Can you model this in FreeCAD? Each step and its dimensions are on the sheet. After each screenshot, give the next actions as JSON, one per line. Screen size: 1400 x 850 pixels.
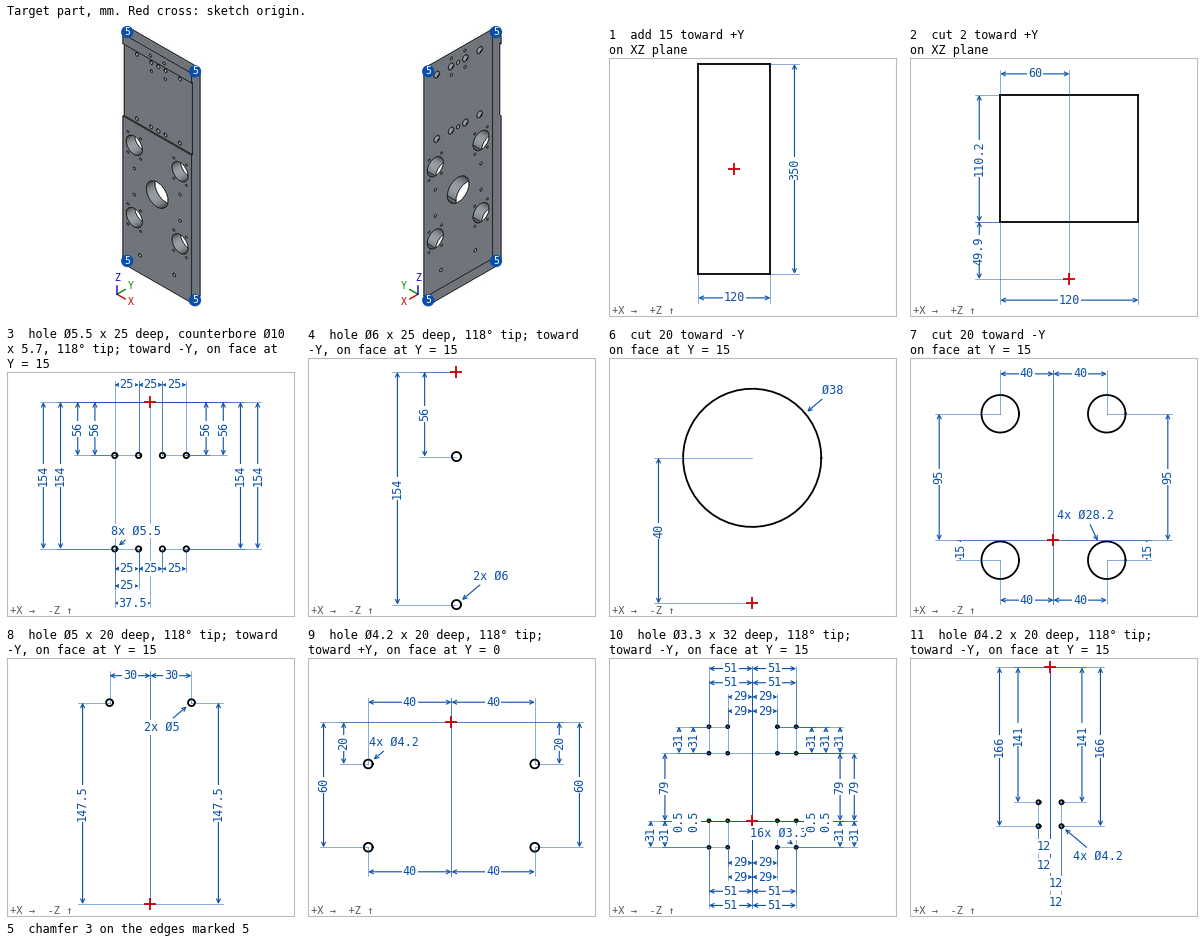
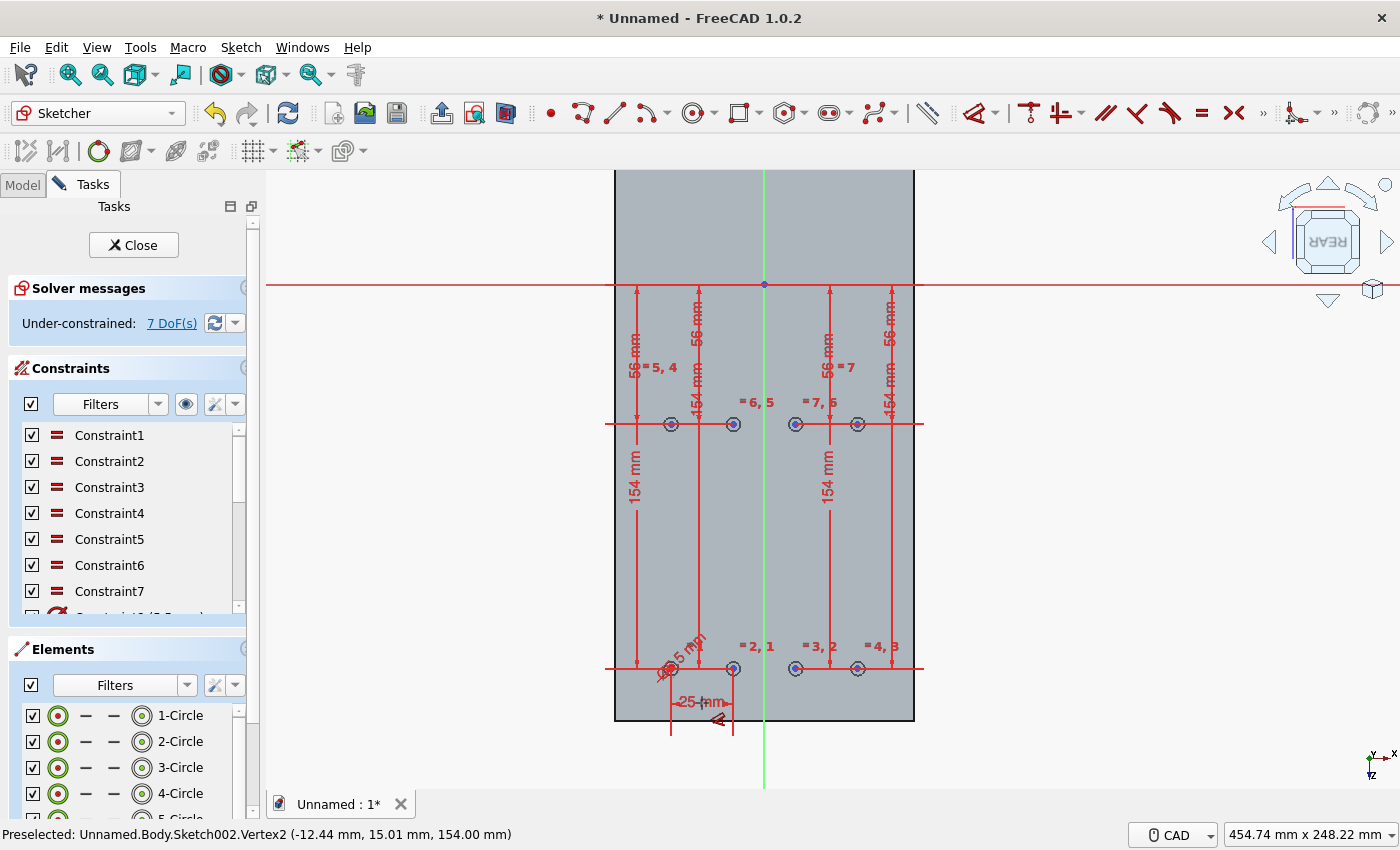
{"action": "left_click", "coordinate": [733, 669]}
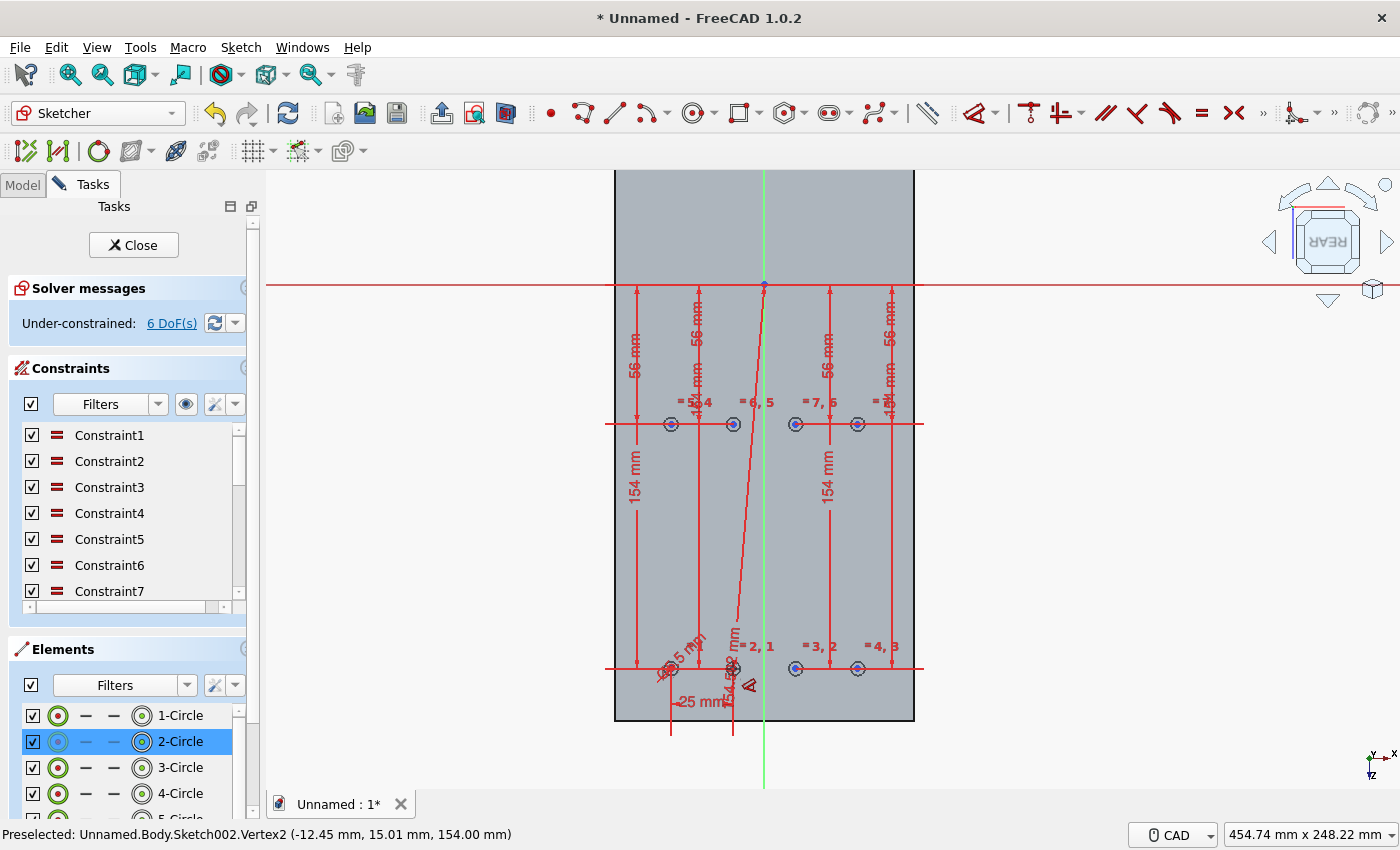
{"action": "left_click", "coordinate": [796, 669]}
{"action": "left_click", "coordinate": [779, 703]}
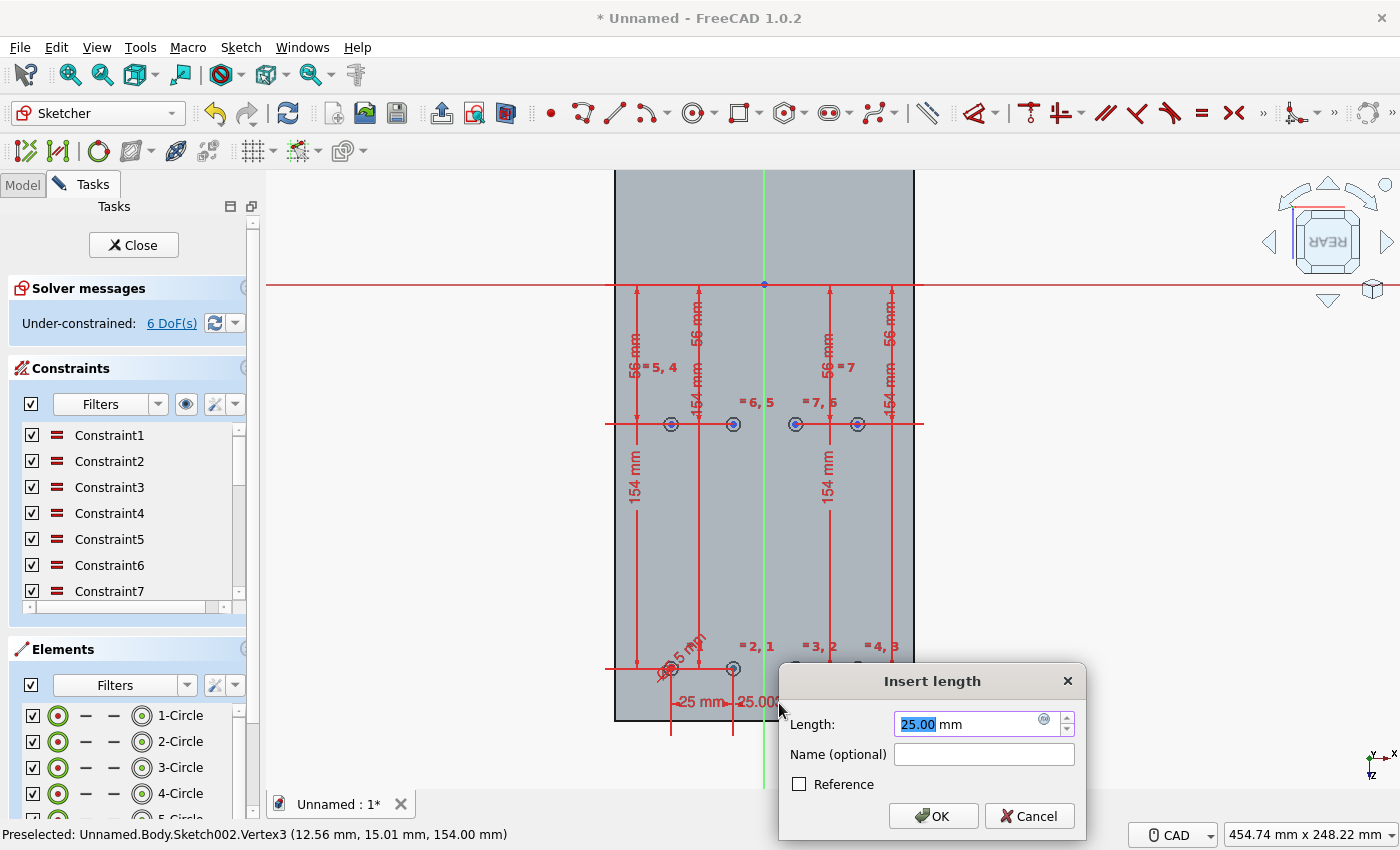
{"action": "type", "text": "25"}
{"action": "key", "text": "Return"}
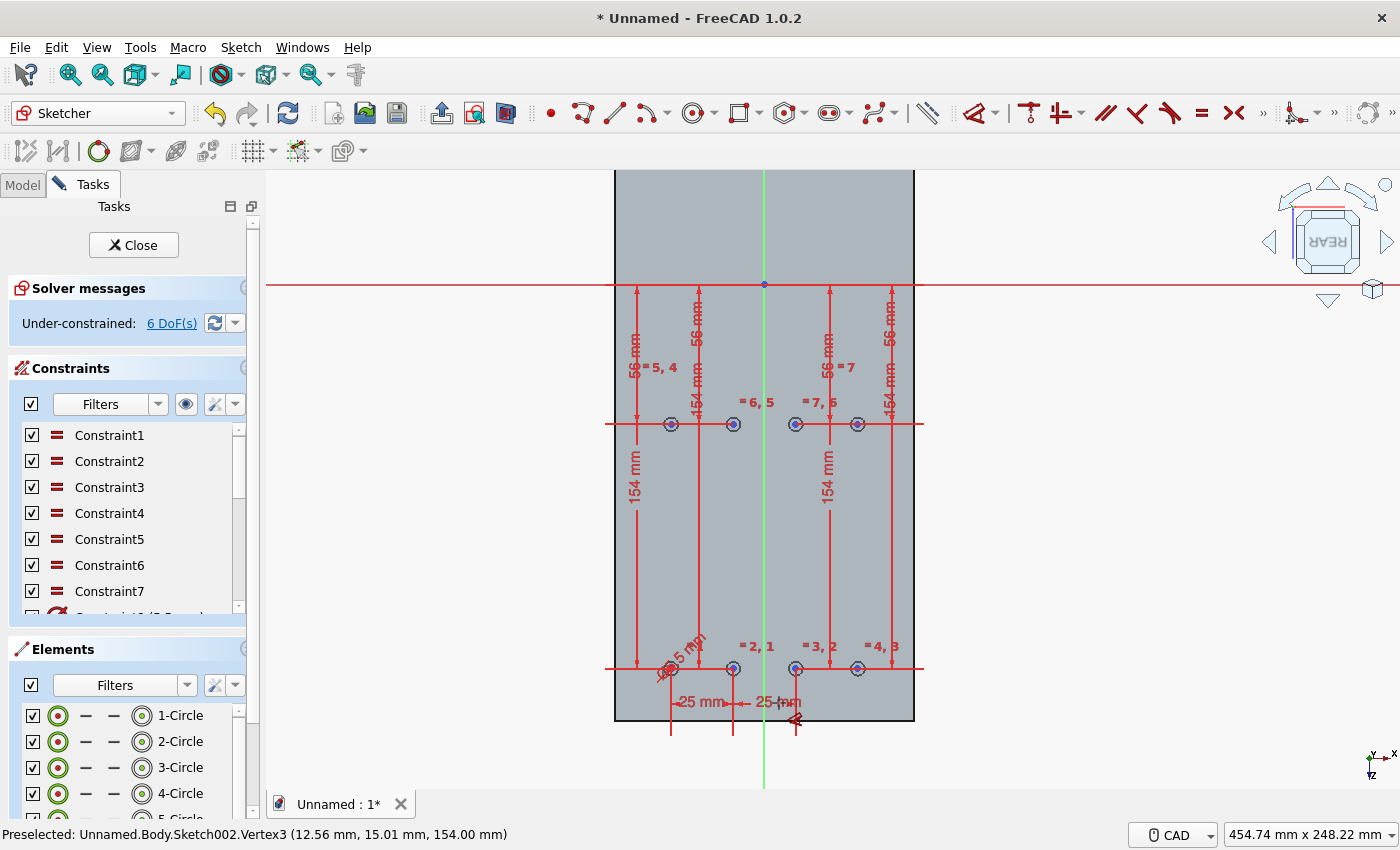
{"action": "left_click", "coordinate": [796, 669]}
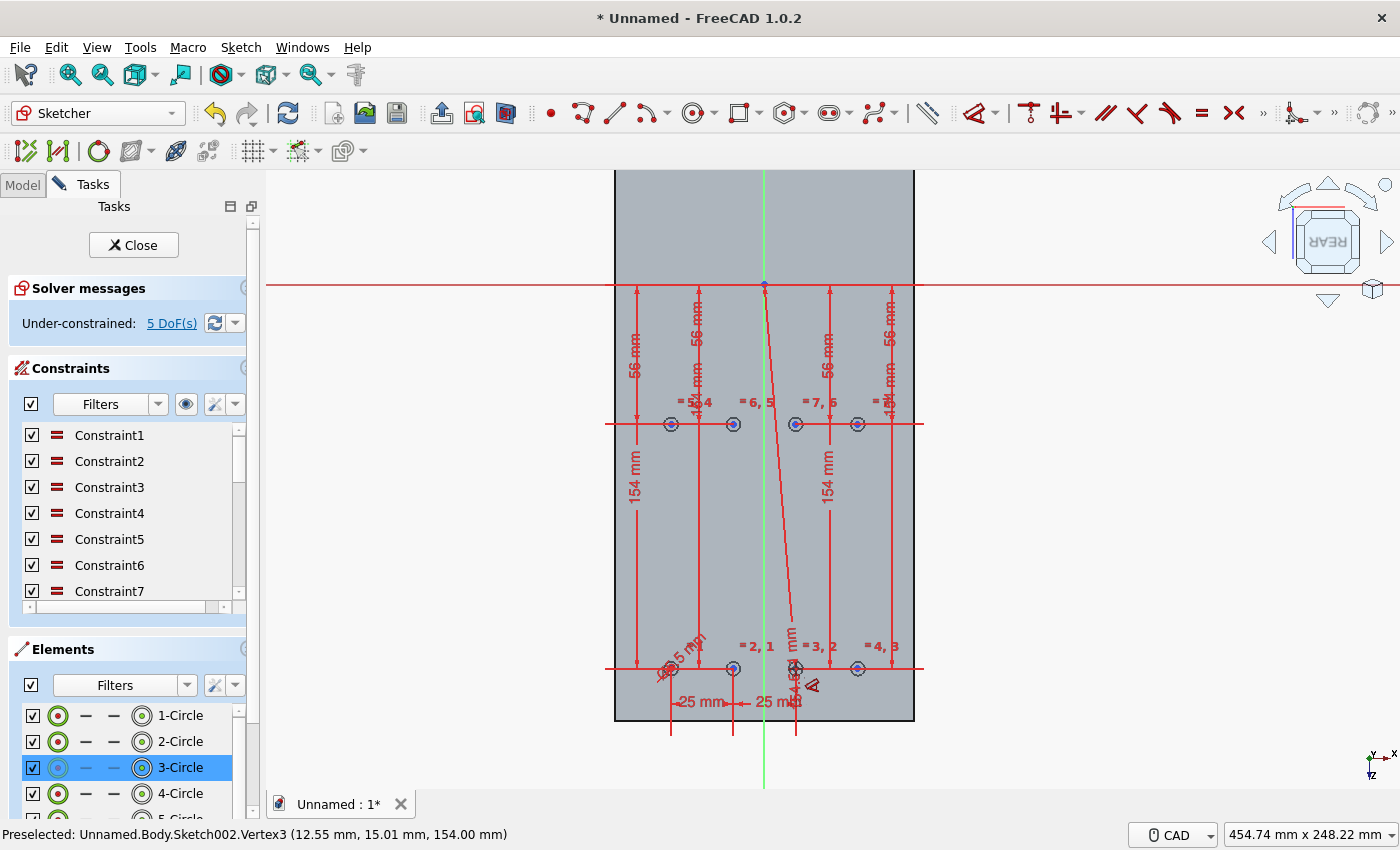
{"action": "left_click", "coordinate": [858, 669]}
{"action": "left_click", "coordinate": [827, 635]}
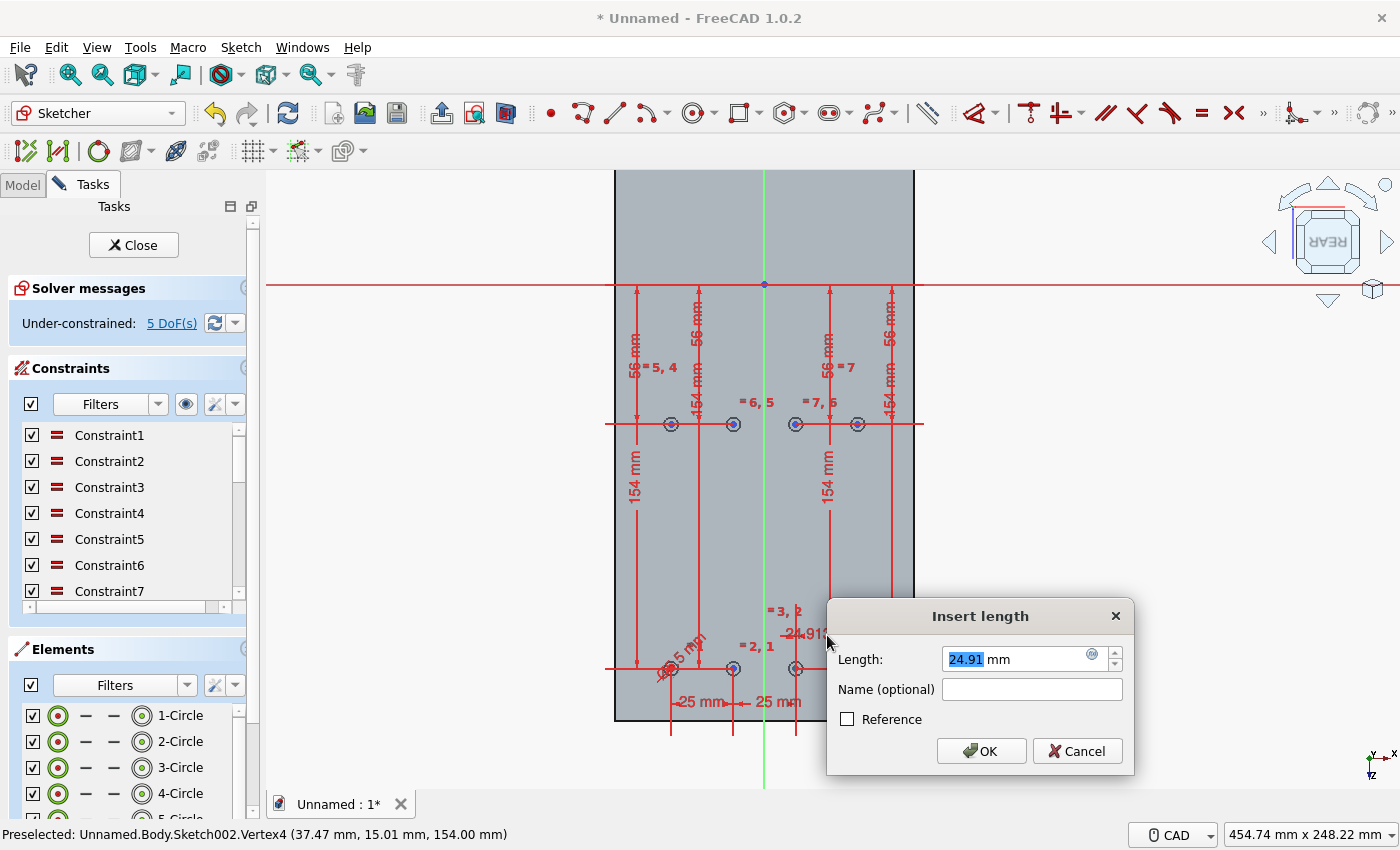
{"action": "type", "text": "25"}
{"action": "key", "text": "Return"}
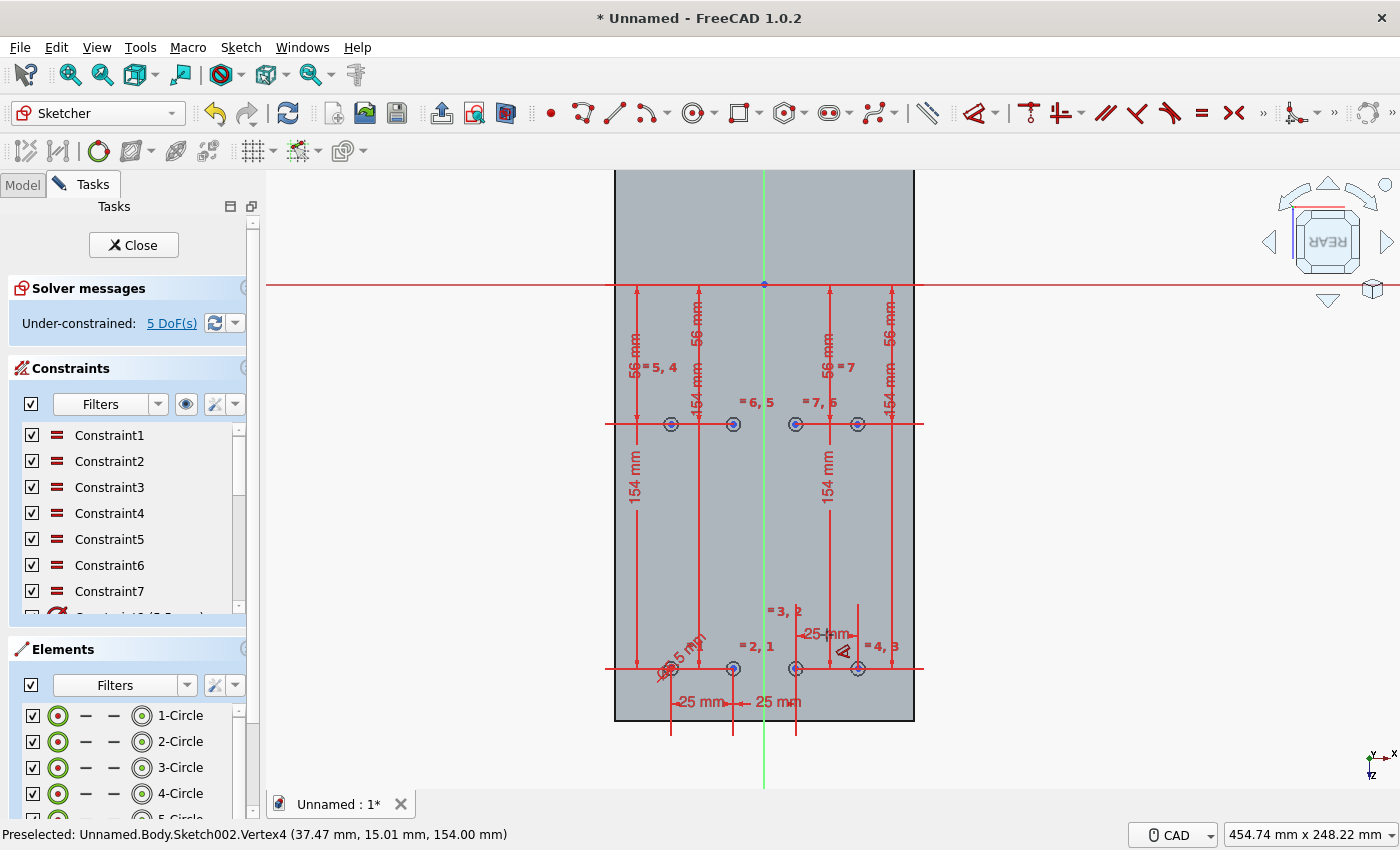
{"action": "left_click", "coordinate": [733, 669]}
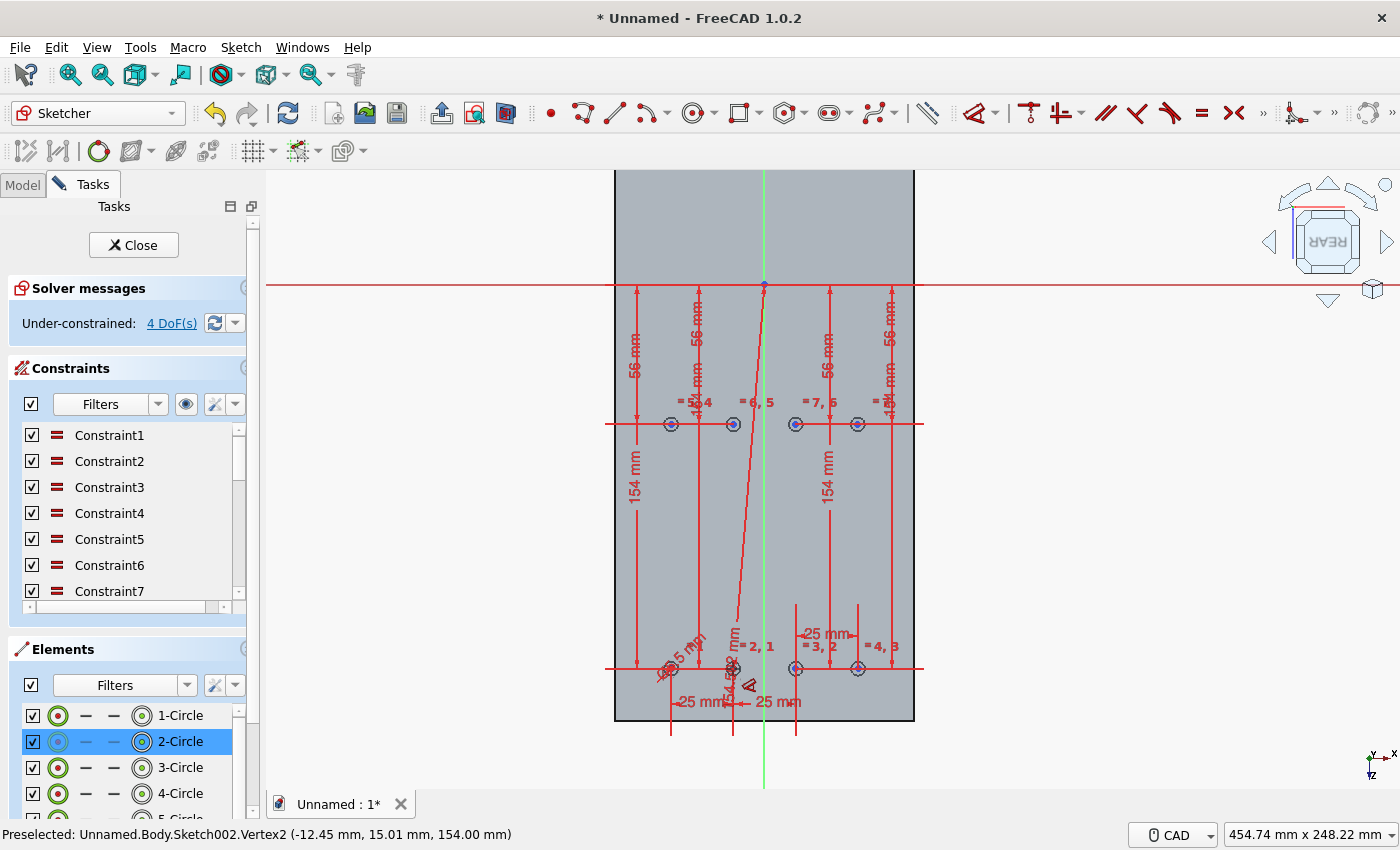
{"action": "left_click", "coordinate": [671, 424]}
{"action": "left_click", "coordinate": [702, 727]}